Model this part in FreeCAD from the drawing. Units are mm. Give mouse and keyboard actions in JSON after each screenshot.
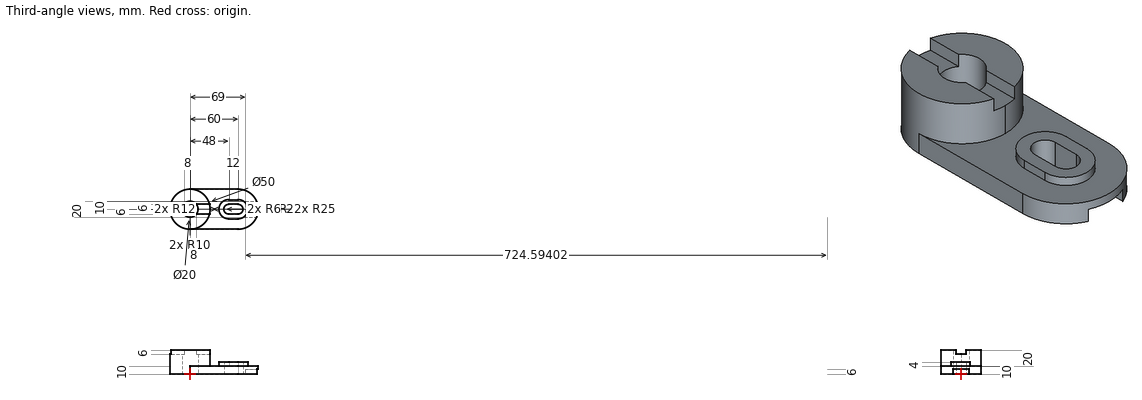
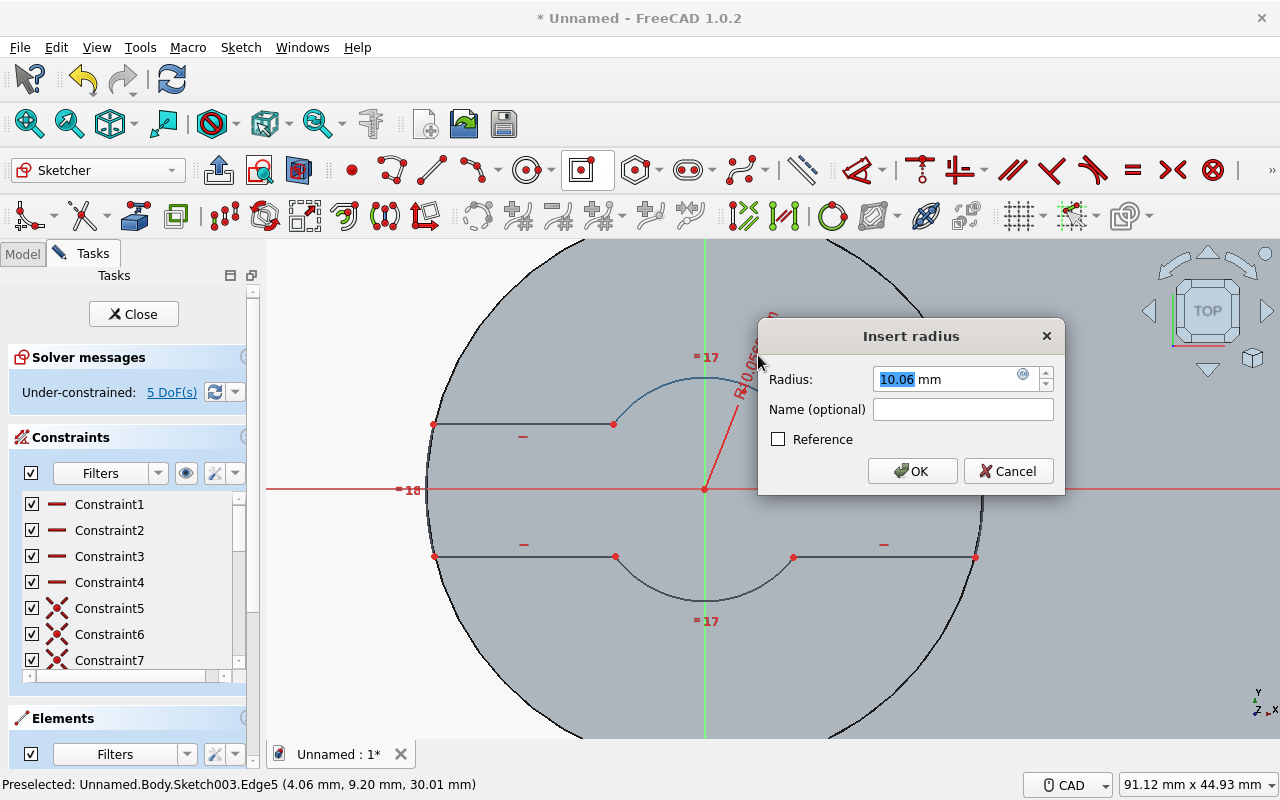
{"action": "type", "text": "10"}
{"action": "key", "text": "Return"}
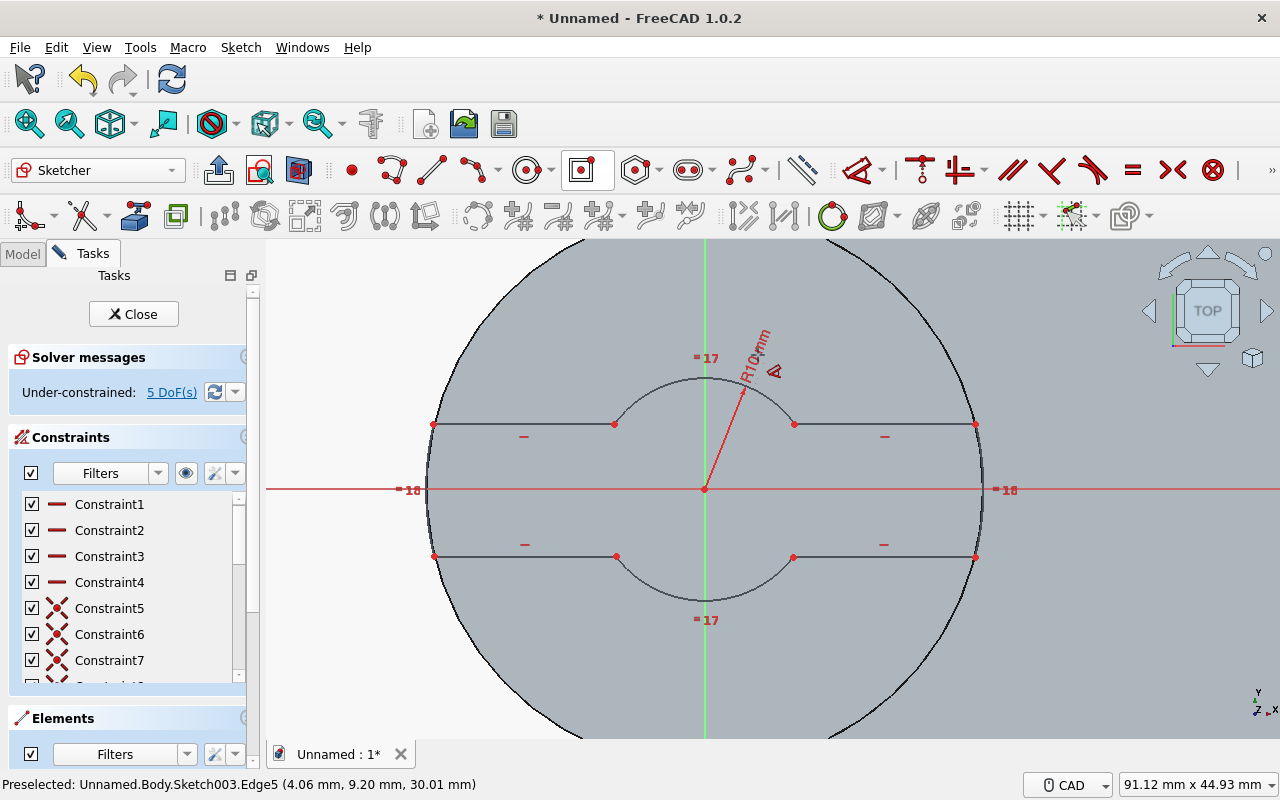
{"action": "left_click", "coordinate": [427, 464]}
{"action": "left_click", "coordinate": [395, 461]}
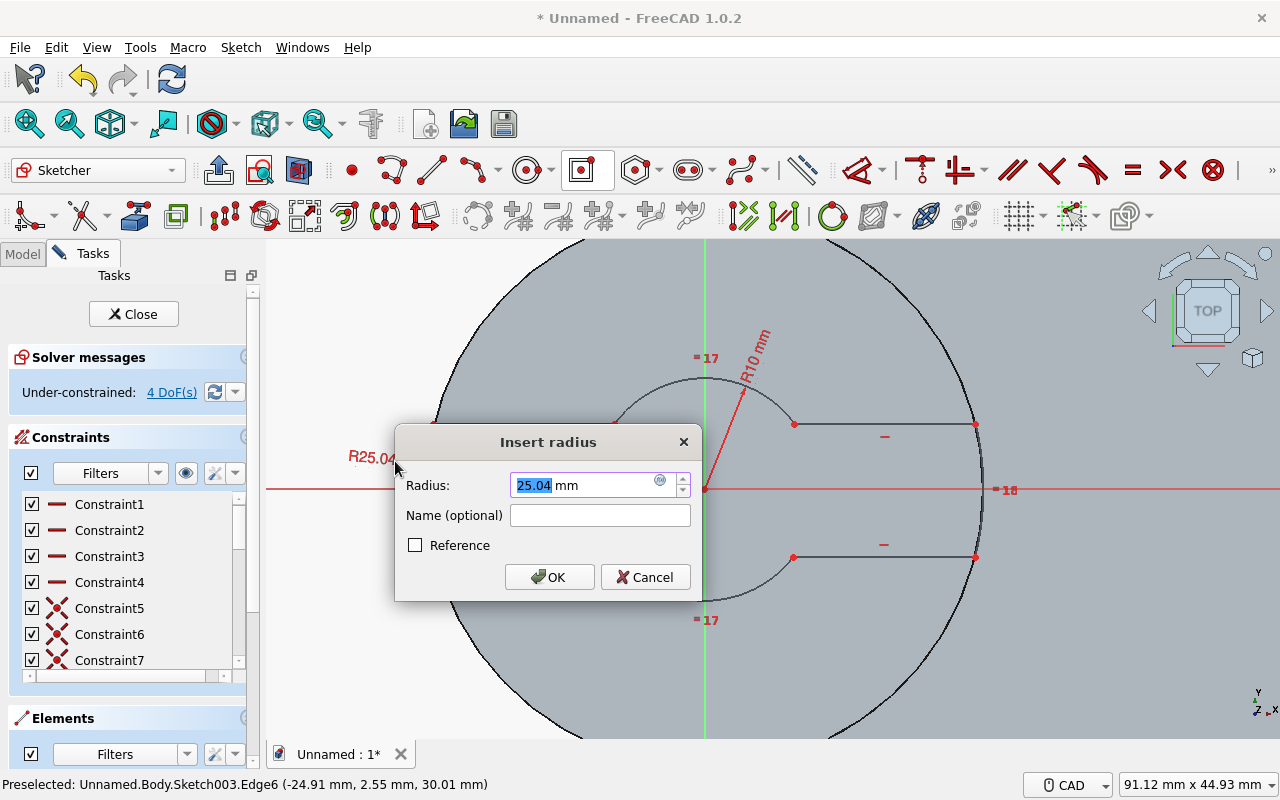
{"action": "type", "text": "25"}
{"action": "key", "text": "Return"}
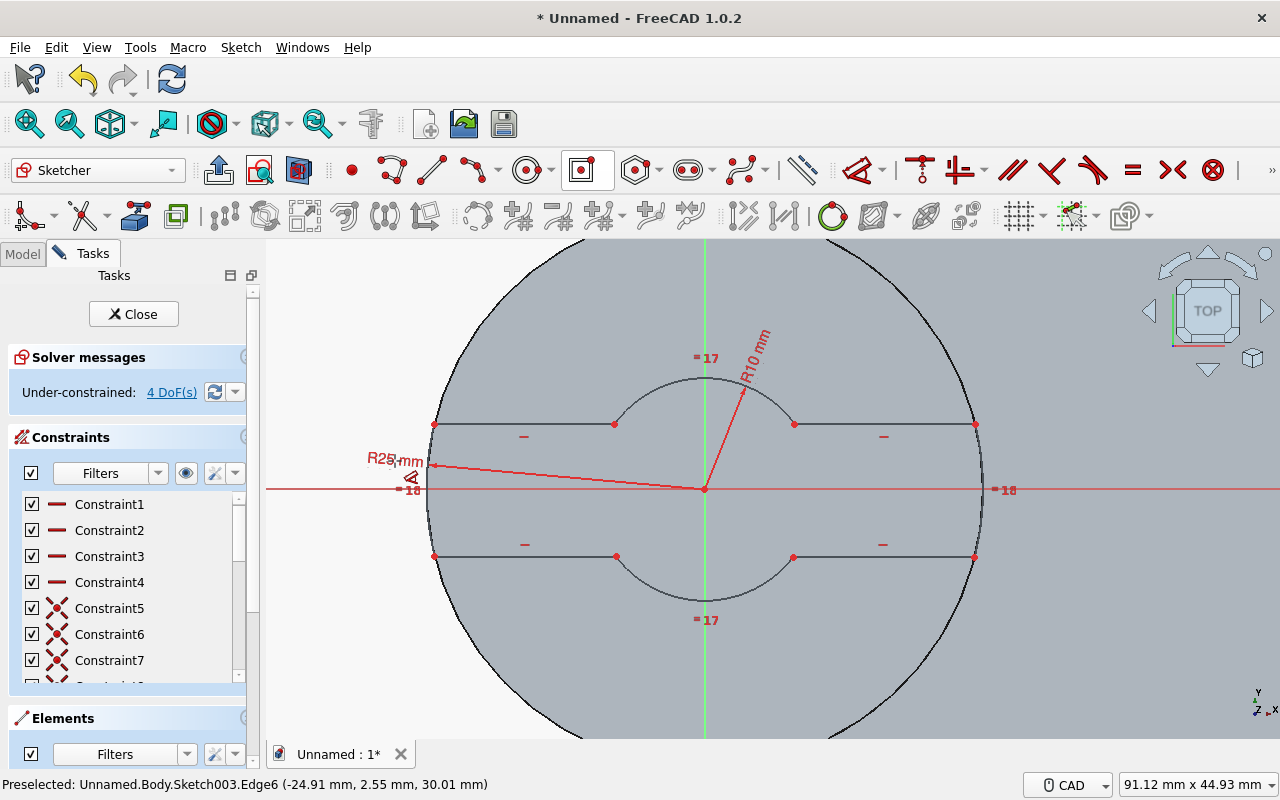
{"action": "left_click", "coordinate": [975, 424]}
{"action": "left_click", "coordinate": [1009, 457]}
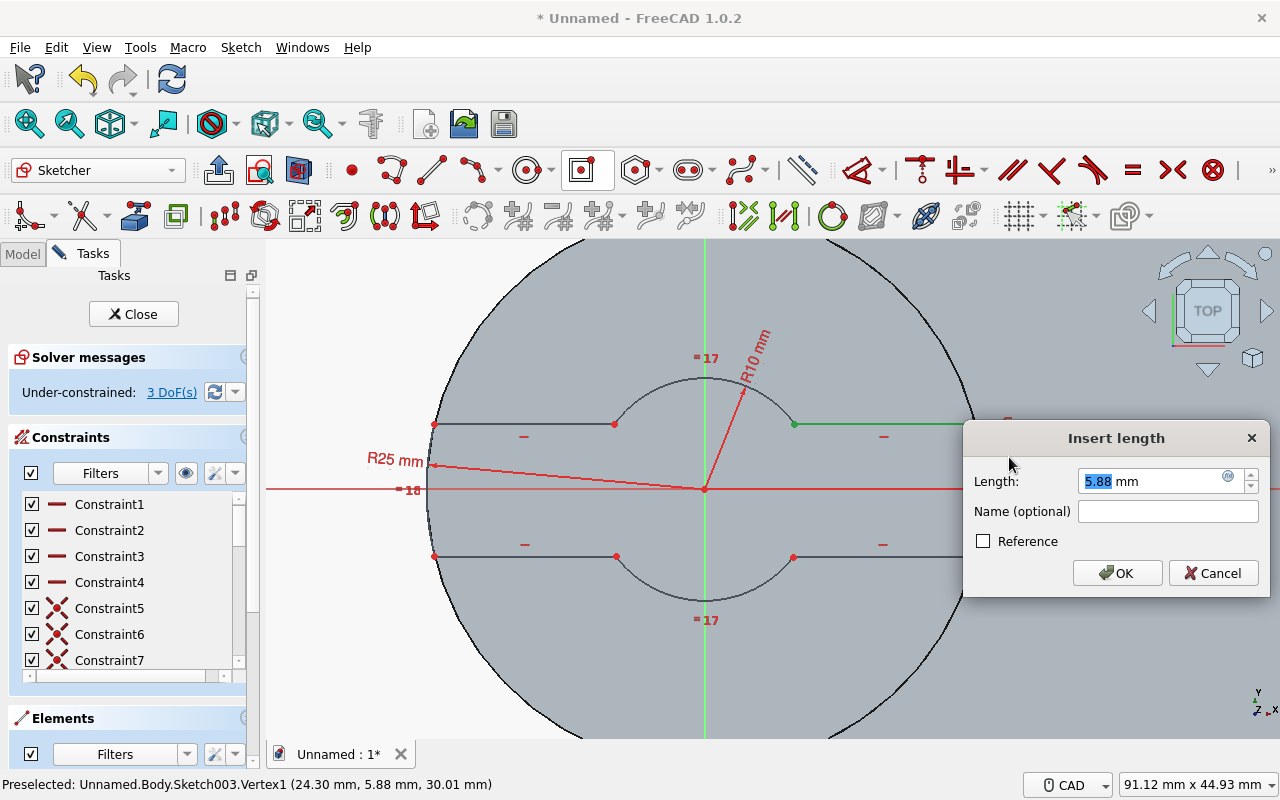
{"action": "type", "text": "6"}
{"action": "key", "text": "Return"}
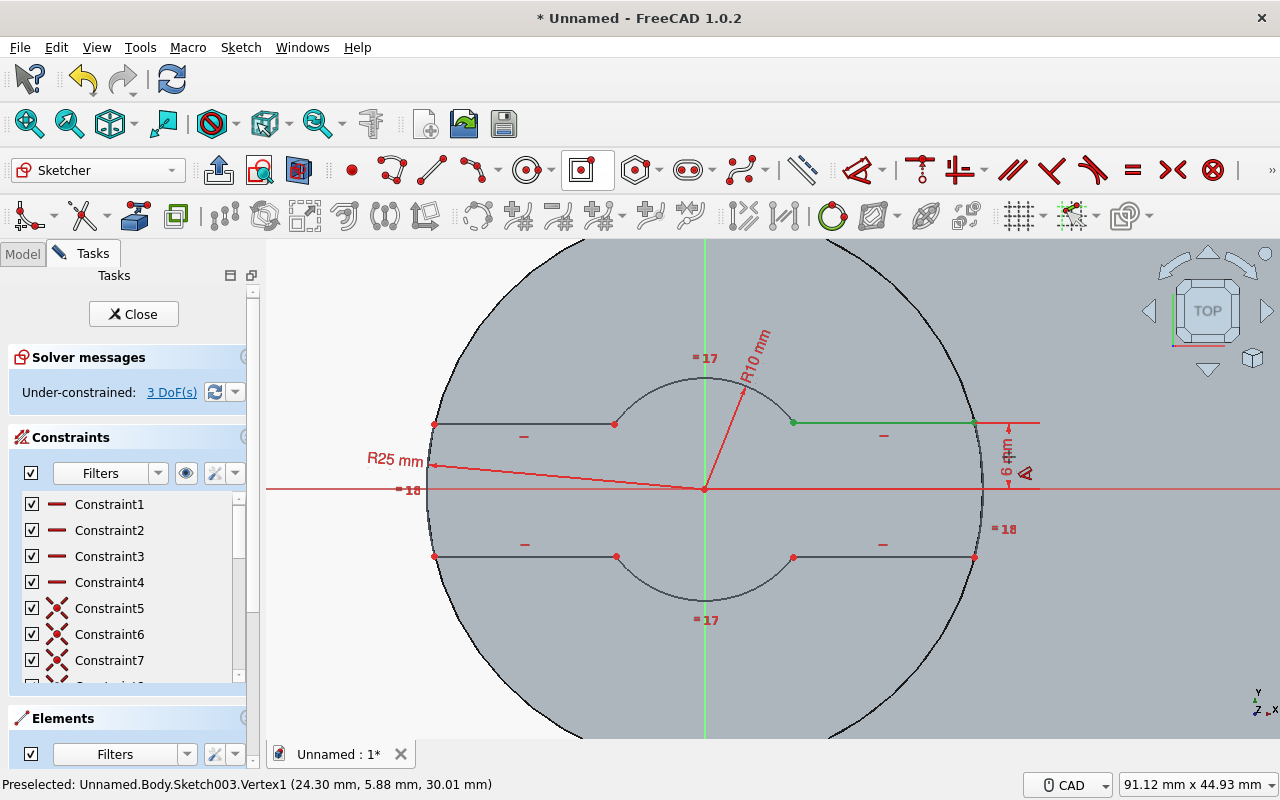
{"action": "left_click", "coordinate": [615, 424]}
{"action": "left_click", "coordinate": [628, 390]}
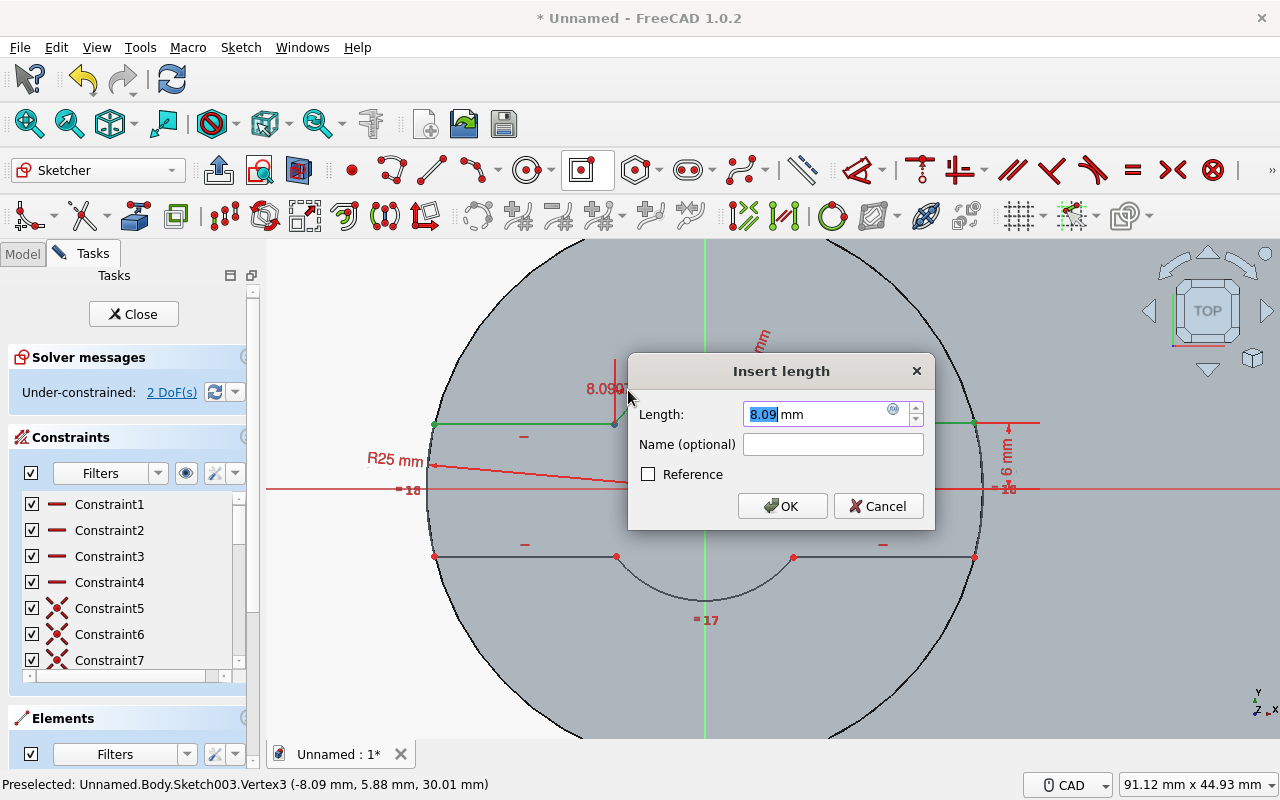
{"action": "type", "text": "8"}
{"action": "key", "text": "Return"}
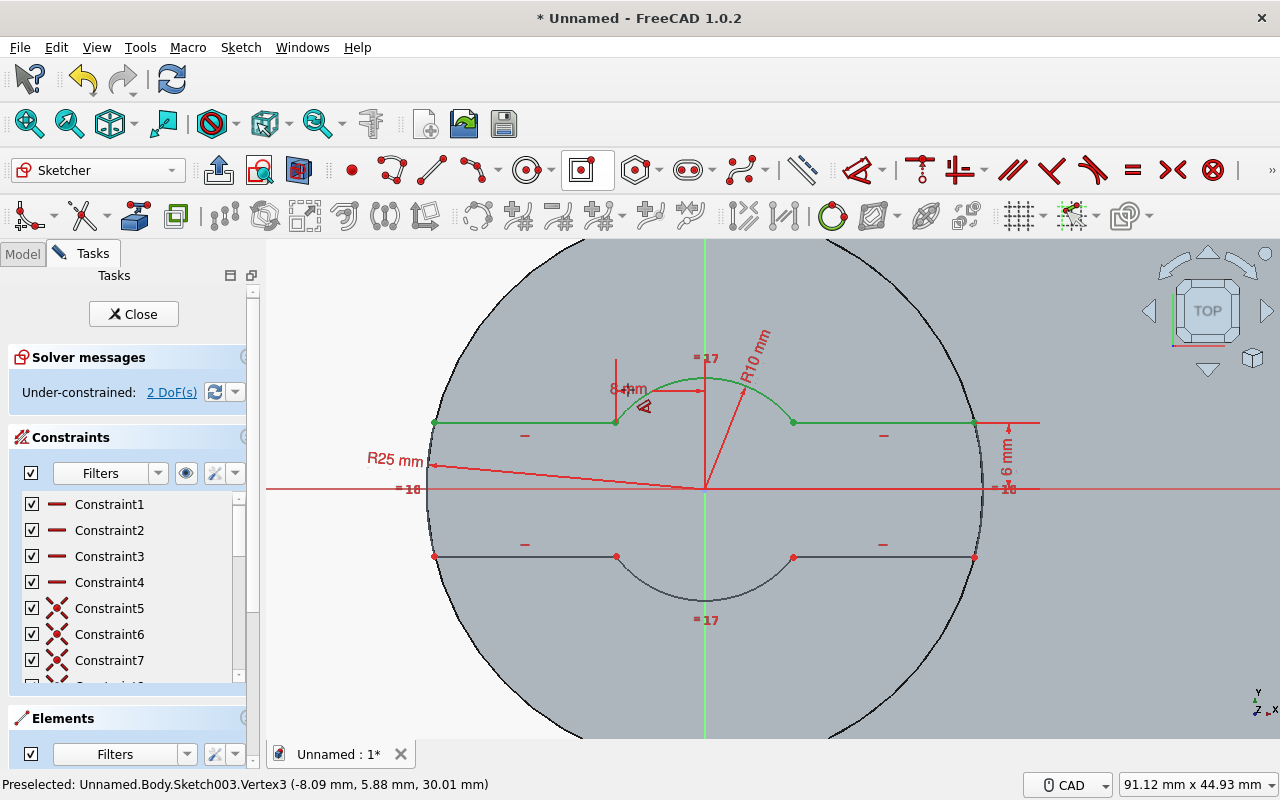
{"action": "left_click", "coordinate": [435, 557]}
{"action": "left_click", "coordinate": [401, 523]}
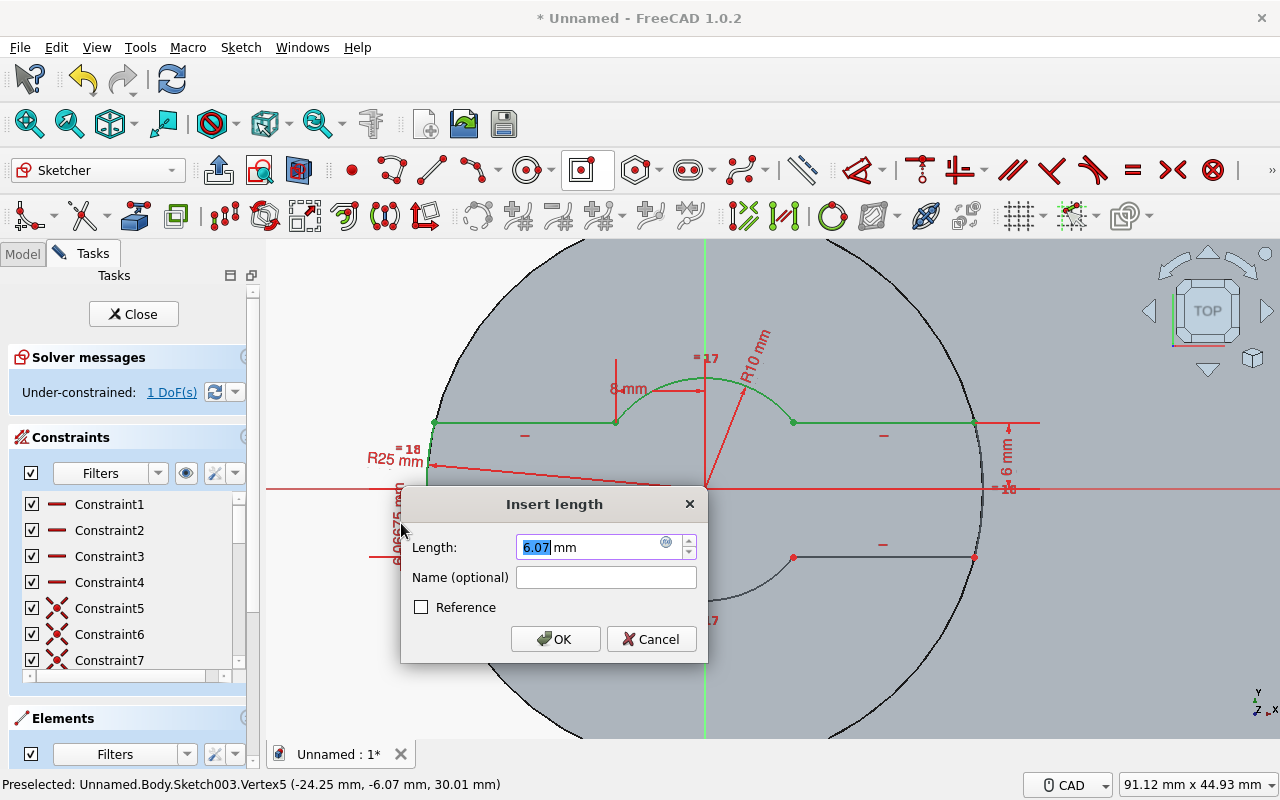
{"action": "type", "text": "6"}
{"action": "key", "text": "Return"}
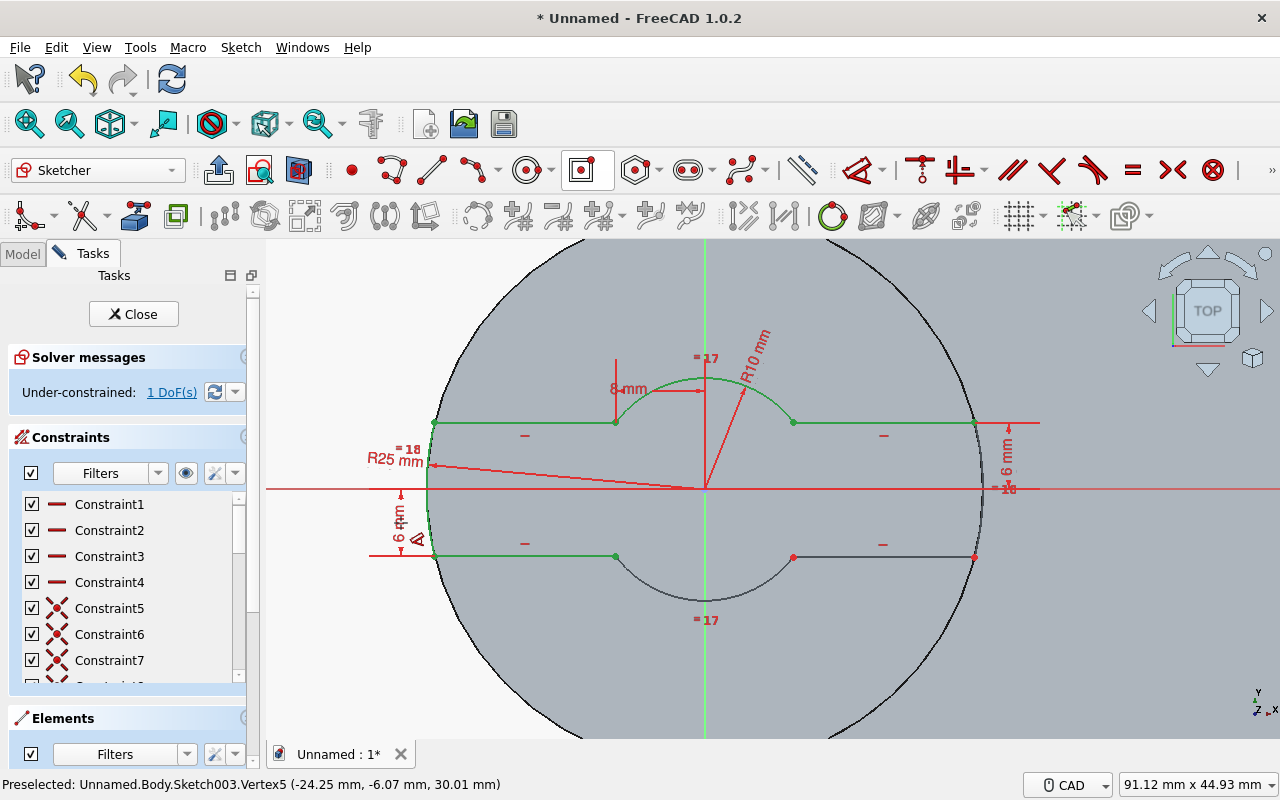
{"action": "left_click", "coordinate": [793, 557]}
{"action": "left_click", "coordinate": [780, 591]}